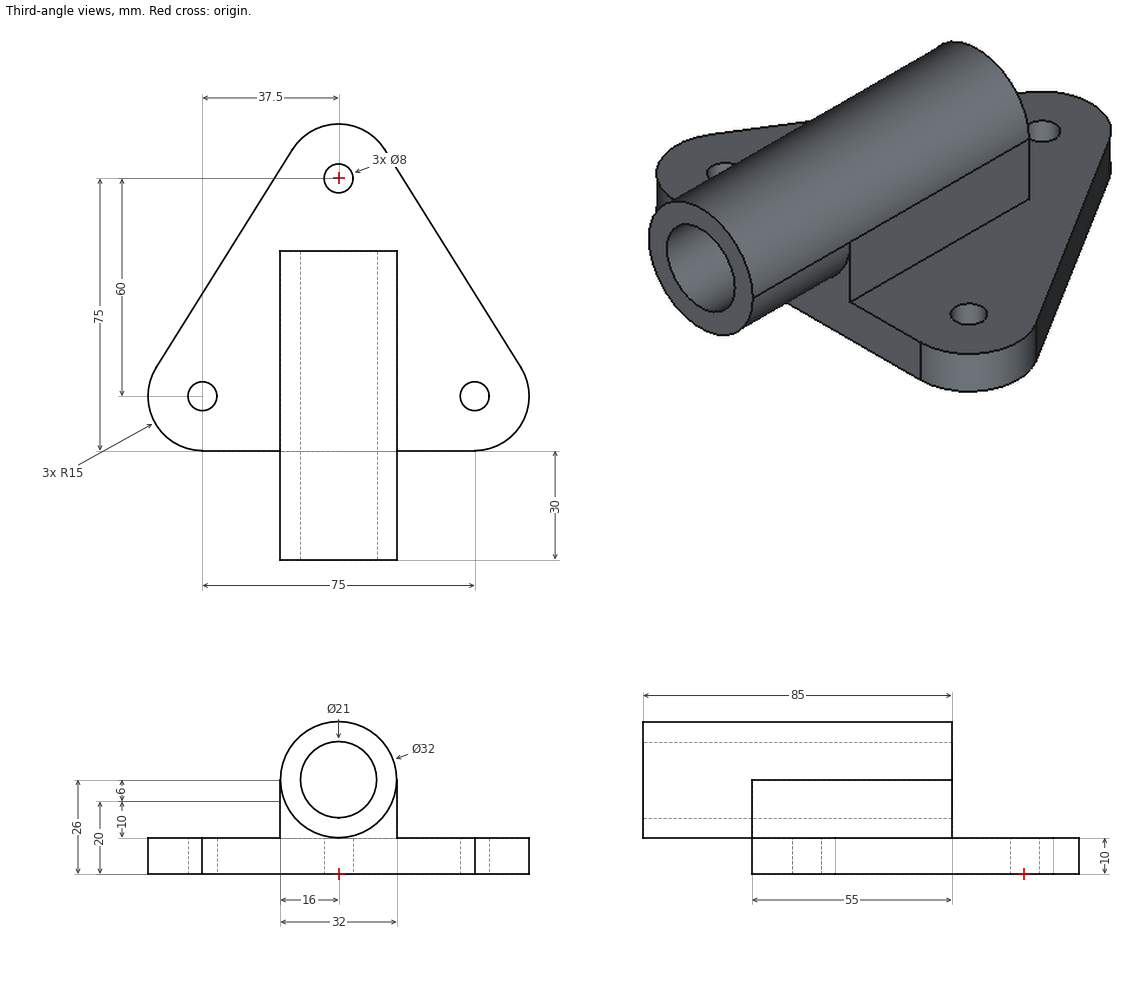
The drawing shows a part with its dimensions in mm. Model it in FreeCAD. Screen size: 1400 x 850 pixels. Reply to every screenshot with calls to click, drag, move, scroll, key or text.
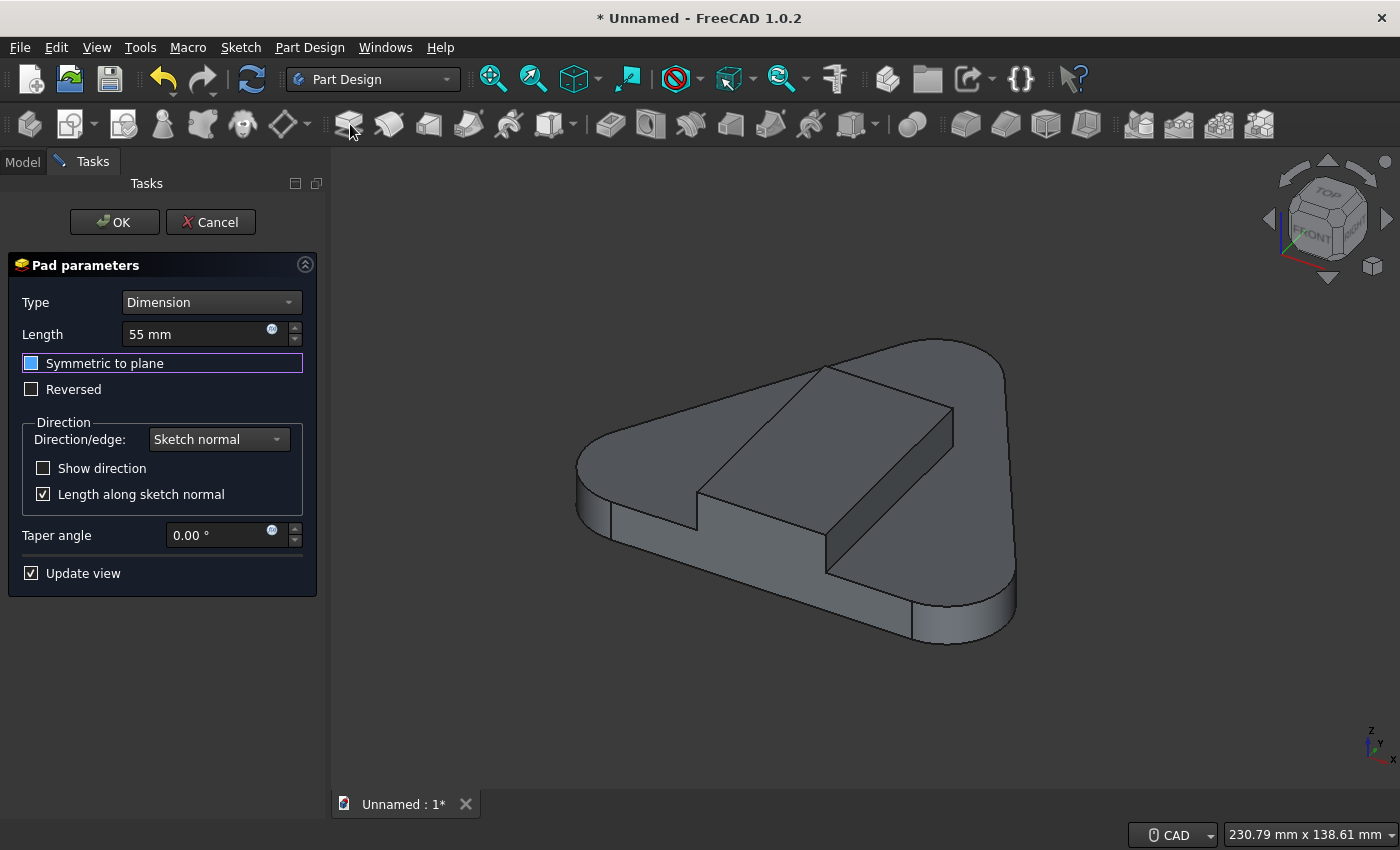
click(30, 389)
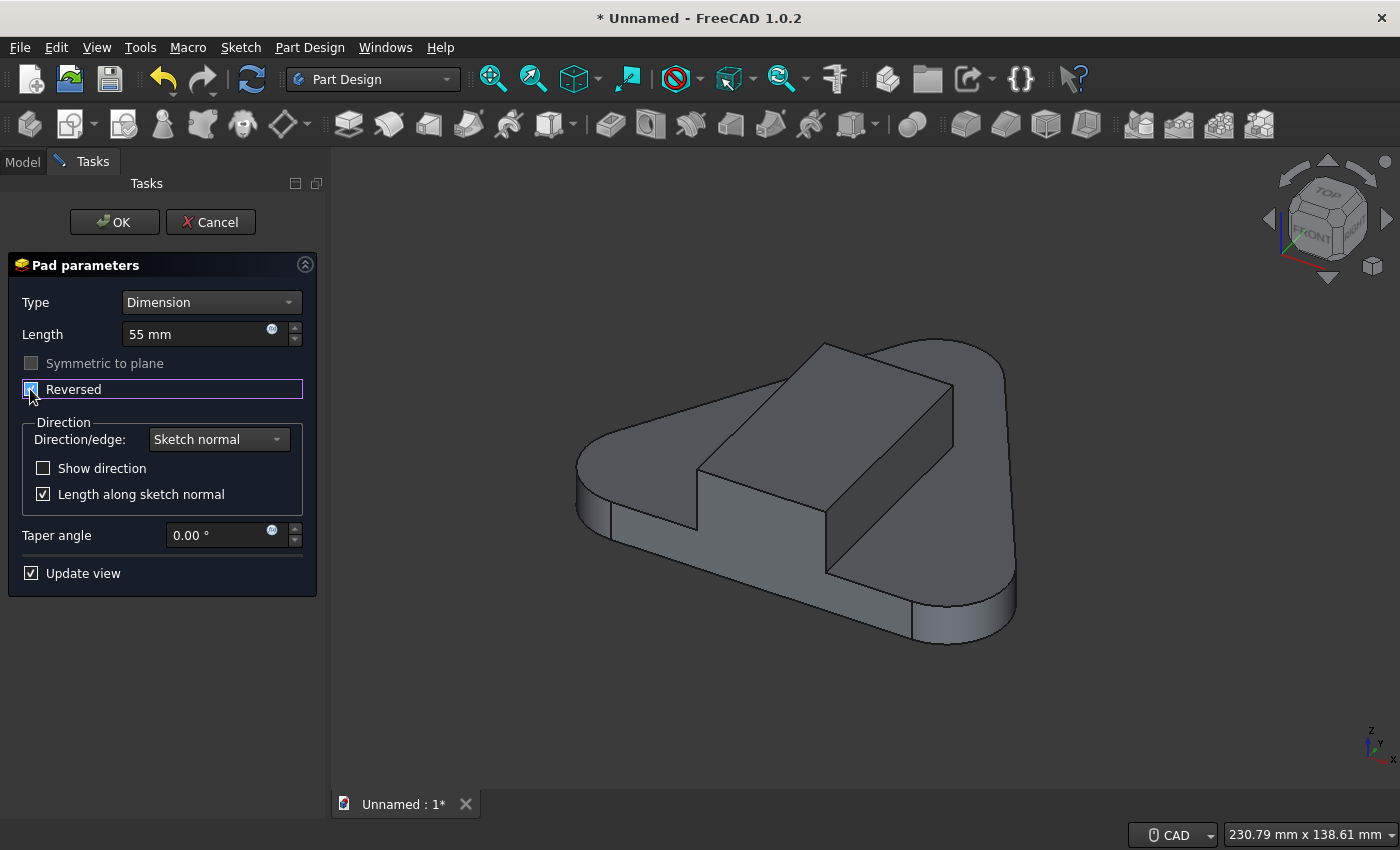
click(115, 222)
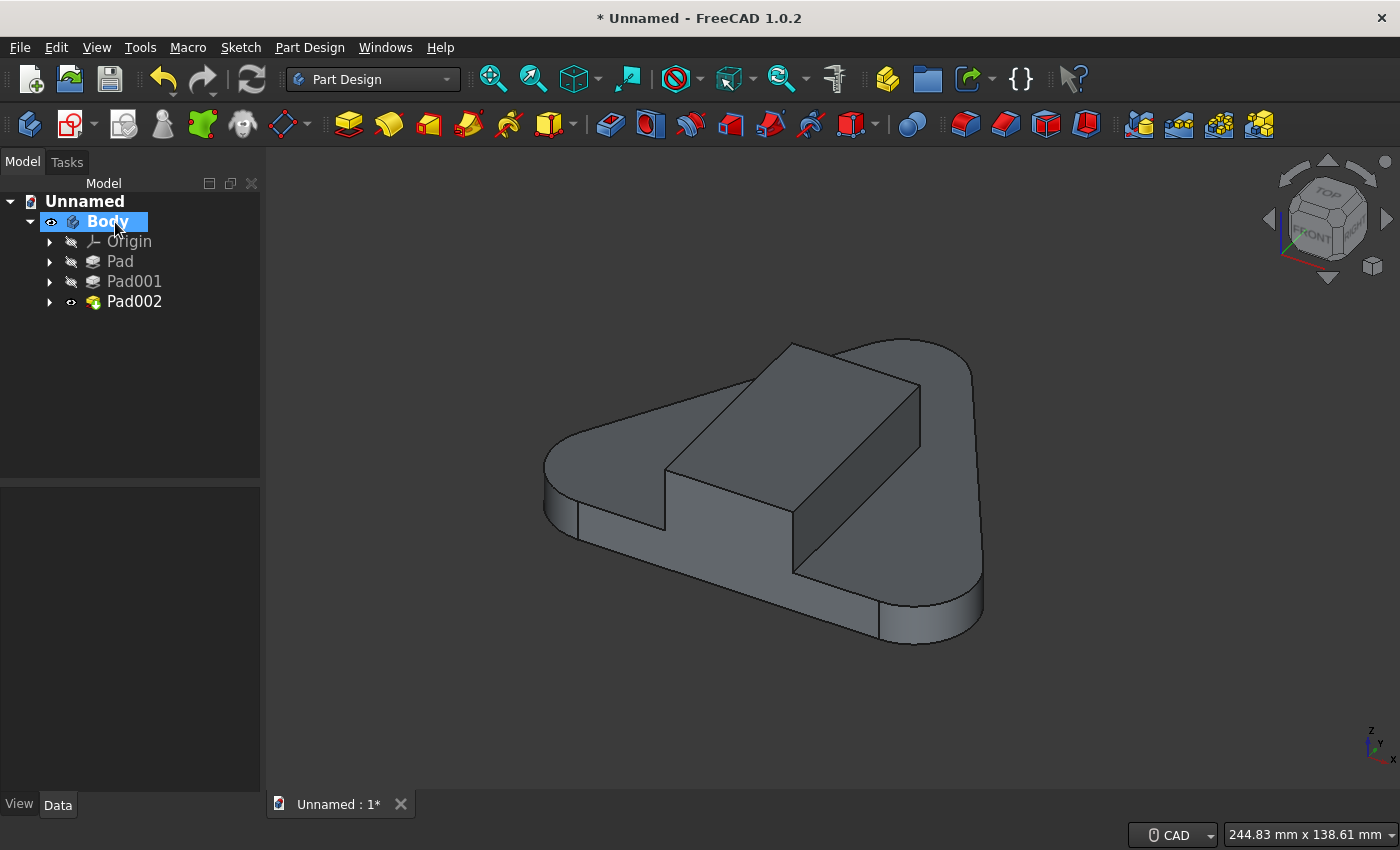
click(729, 539)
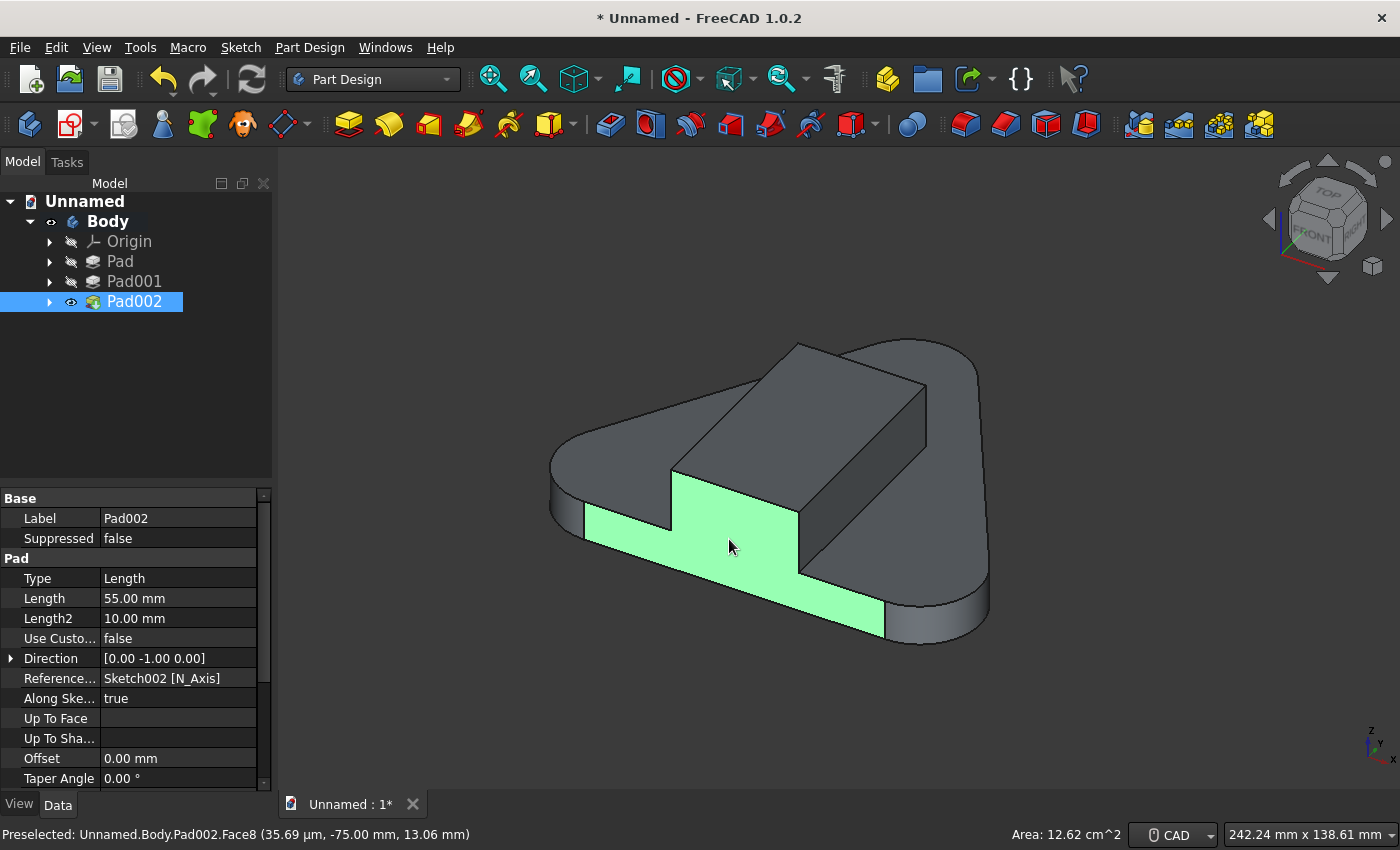
click(70, 124)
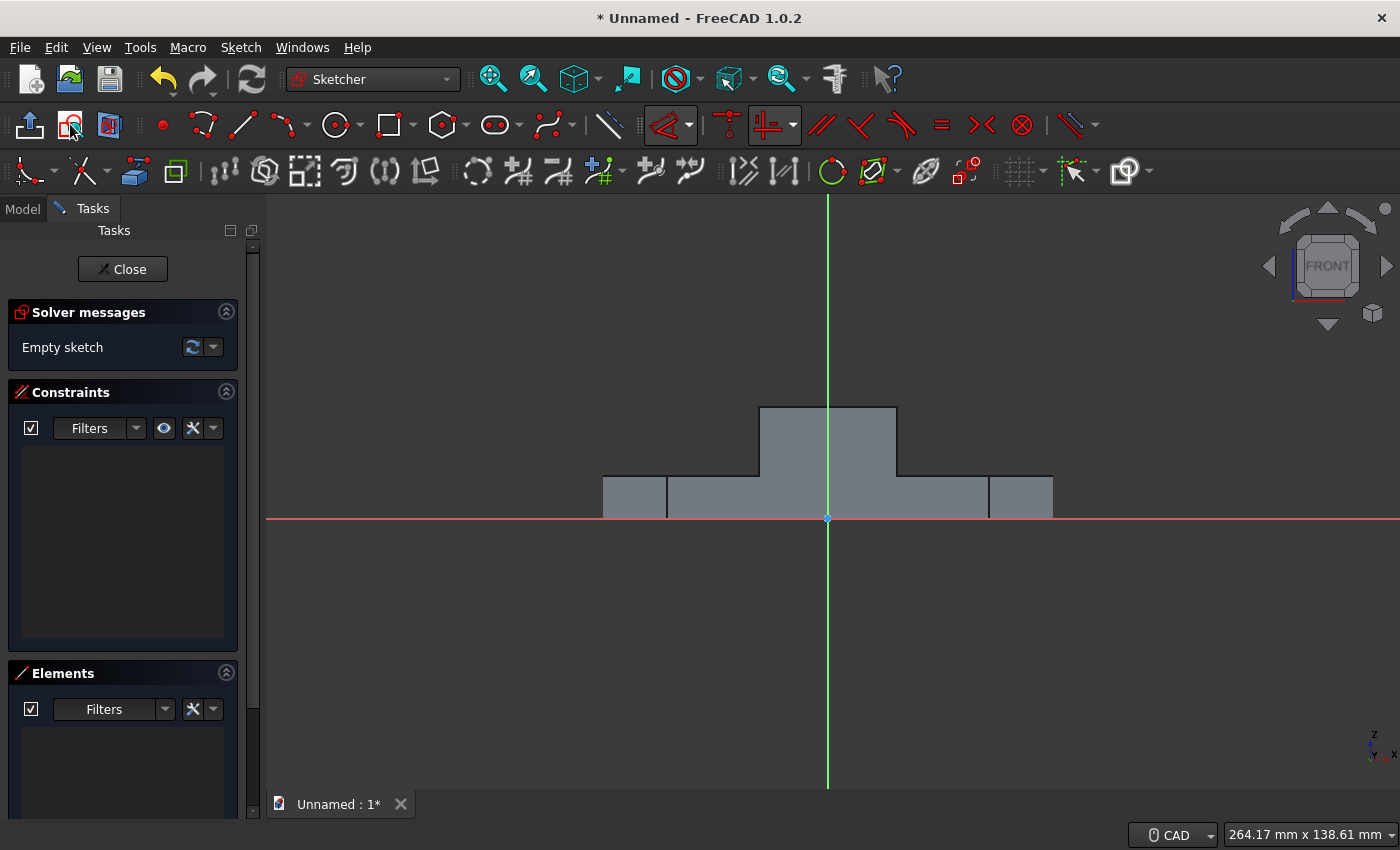
scroll(880, 378, up, 4)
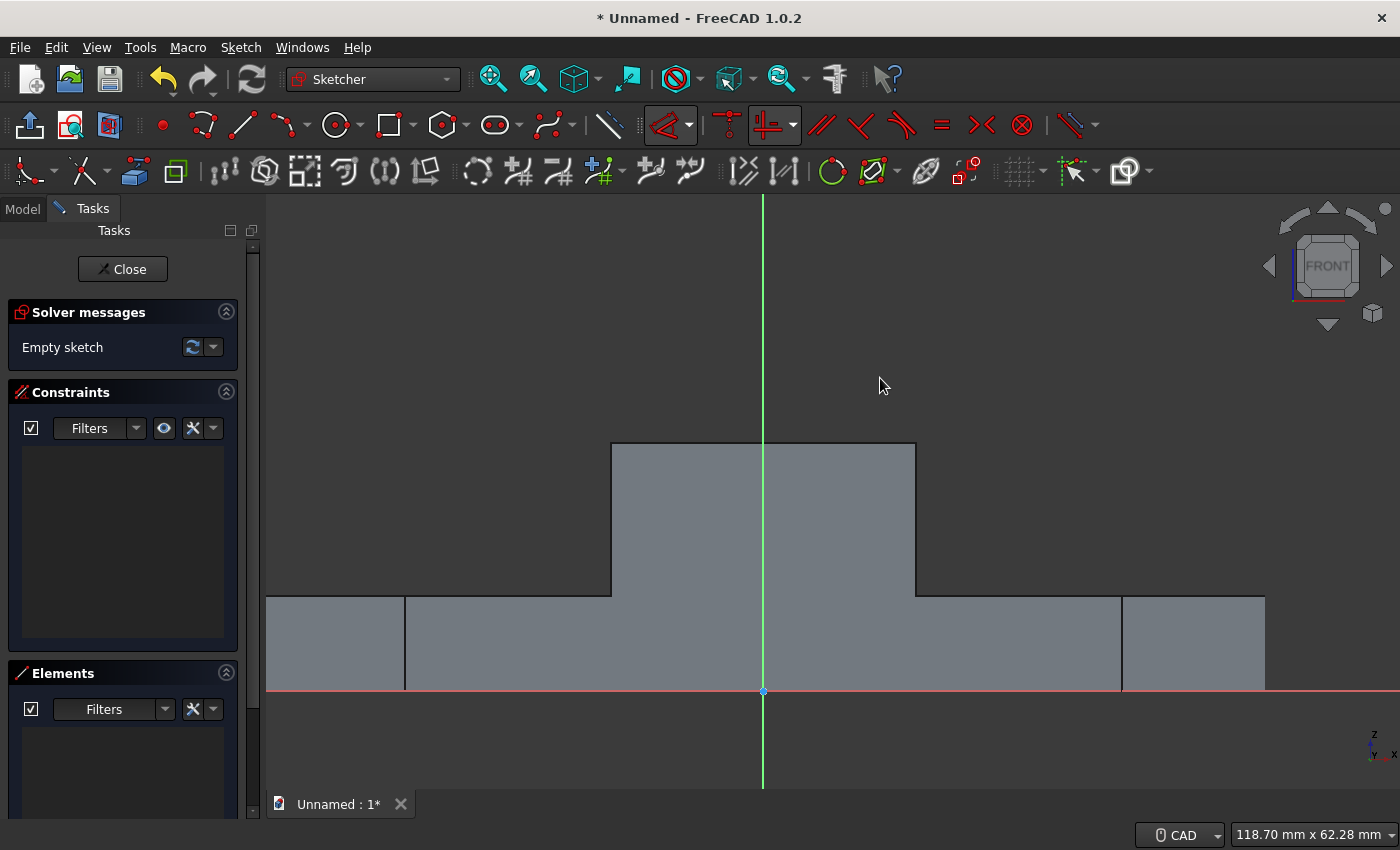
click(336, 126)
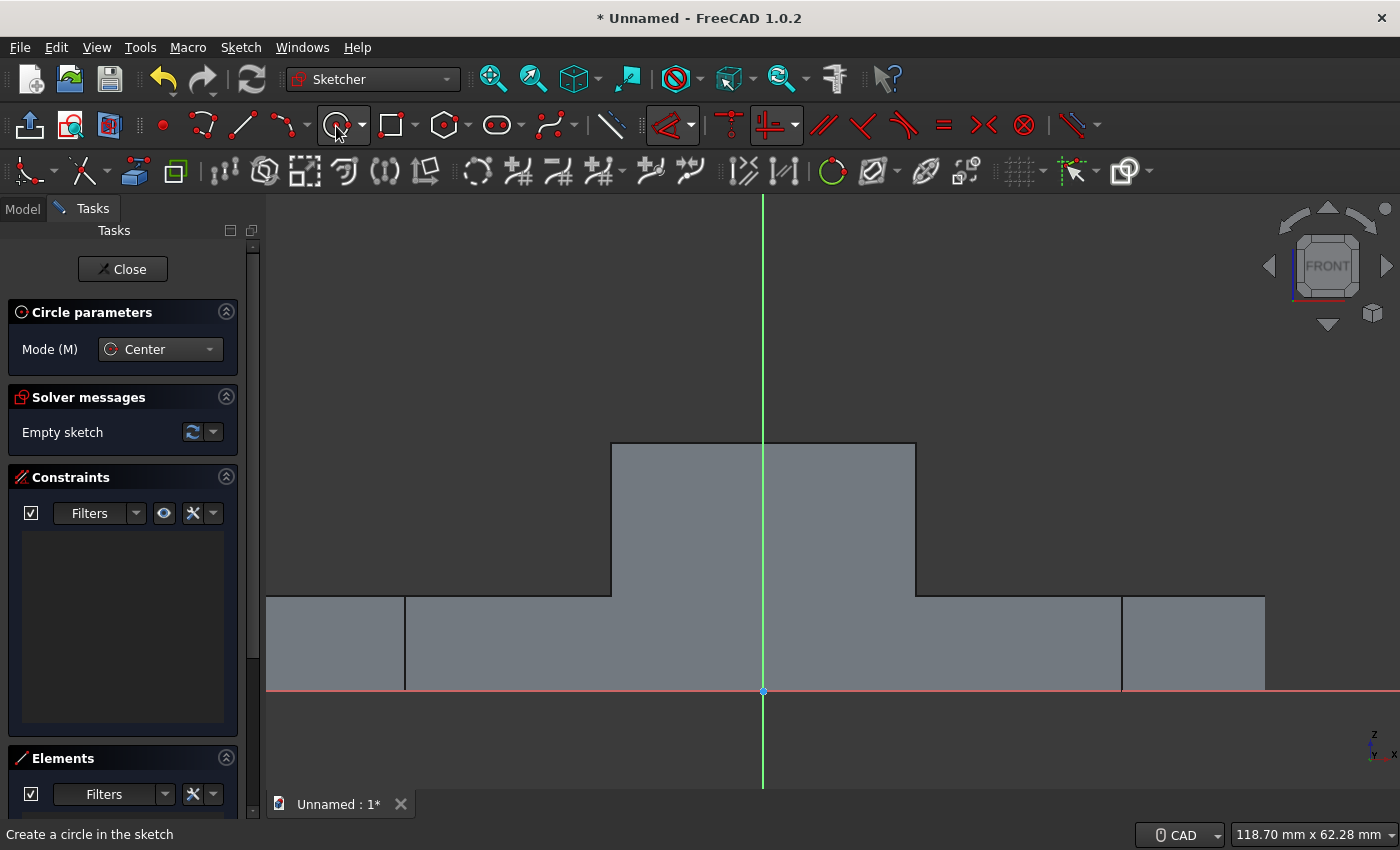
click(763, 443)
click(872, 335)
key(Escape)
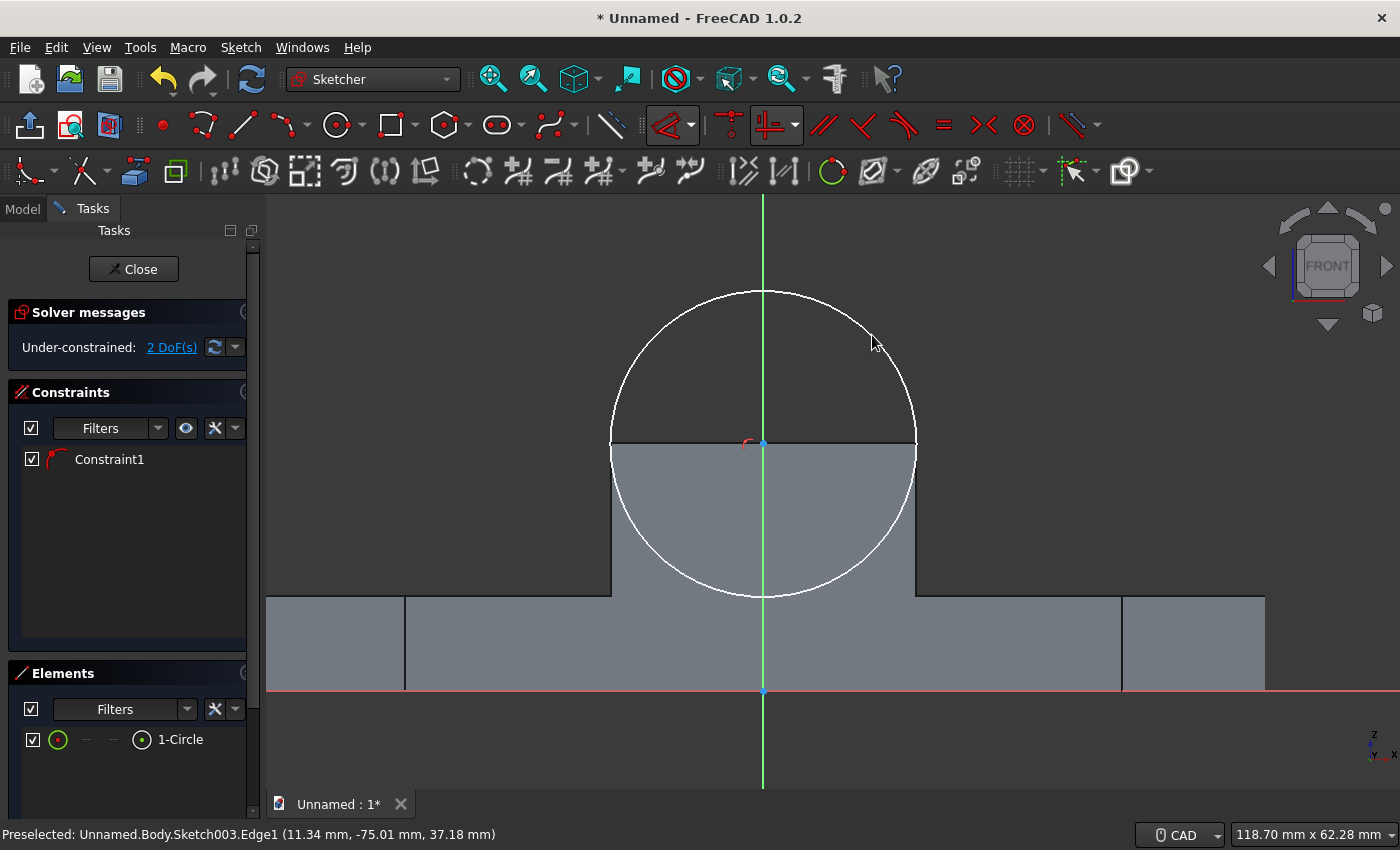
click(871, 335)